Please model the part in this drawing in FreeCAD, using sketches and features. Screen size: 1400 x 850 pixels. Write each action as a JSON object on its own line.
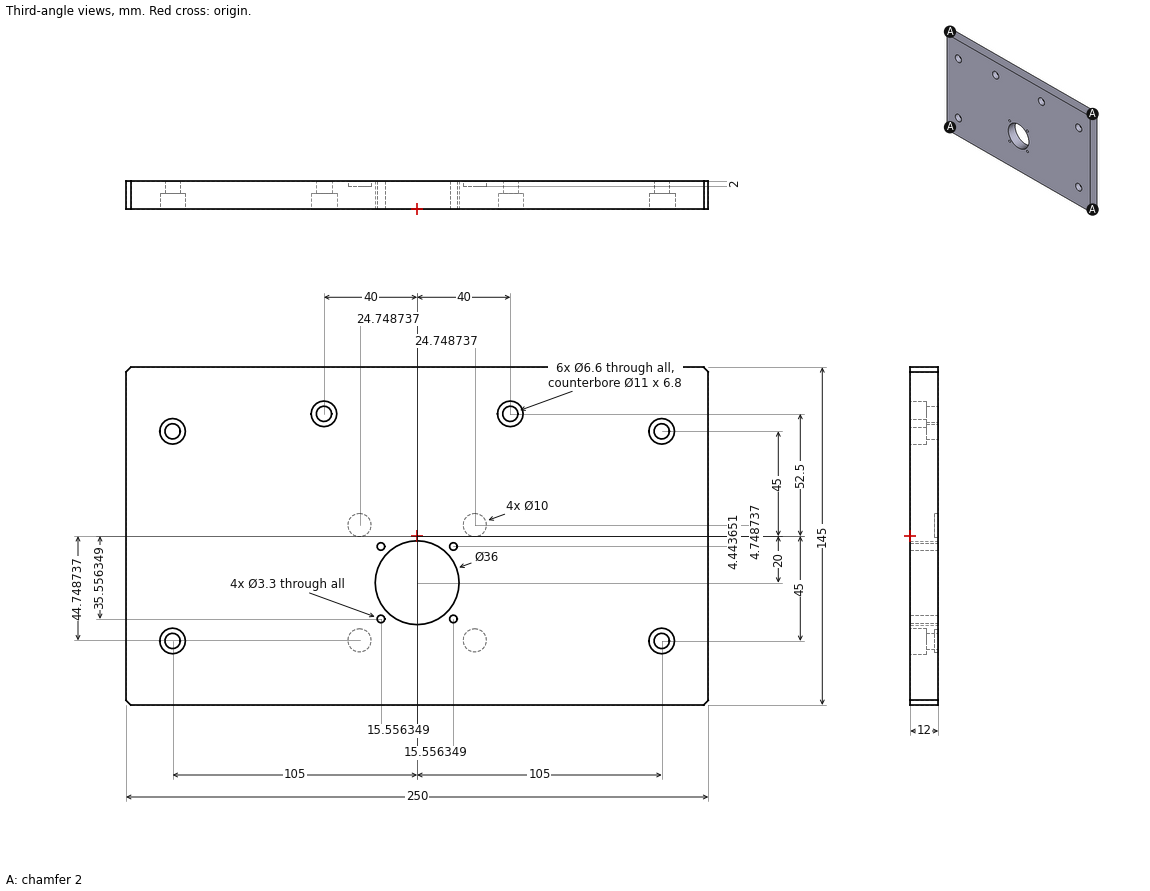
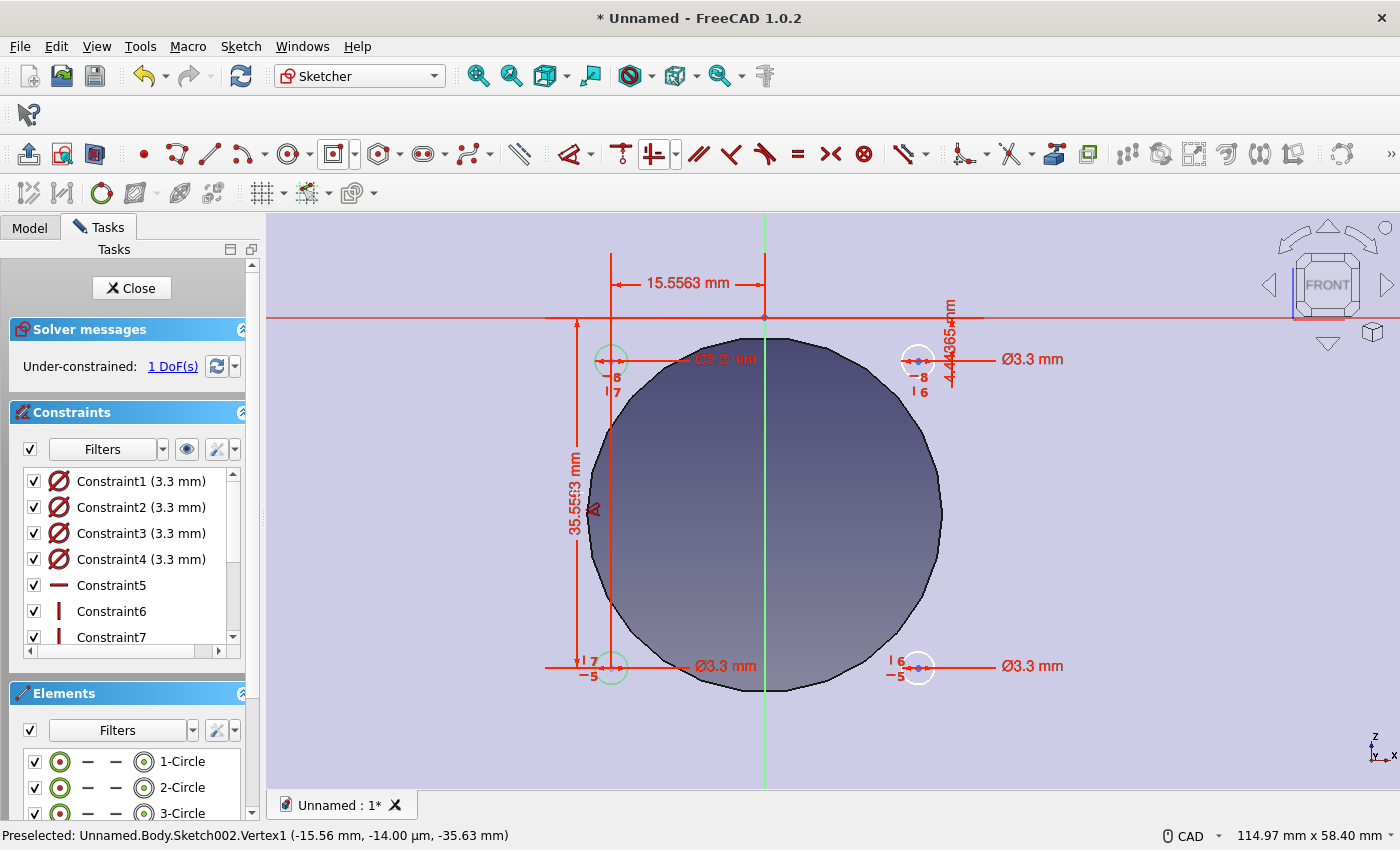
{"action": "left_click", "coordinate": [918, 668]}
{"action": "left_click", "coordinate": [841, 284]}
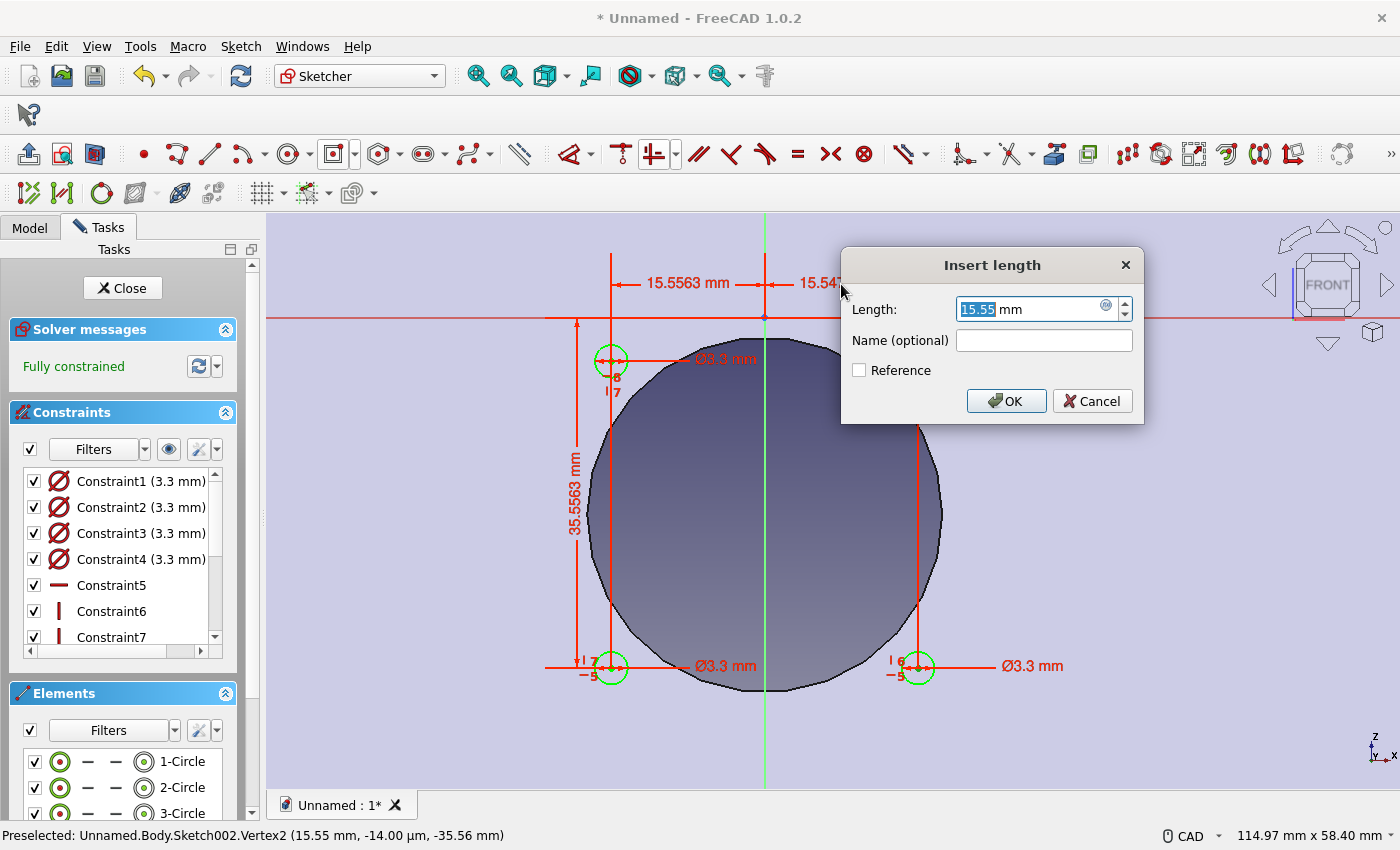
{"action": "type", "text": "15.556349"}
{"action": "key", "text": "Return"}
{"action": "key", "text": "Escape"}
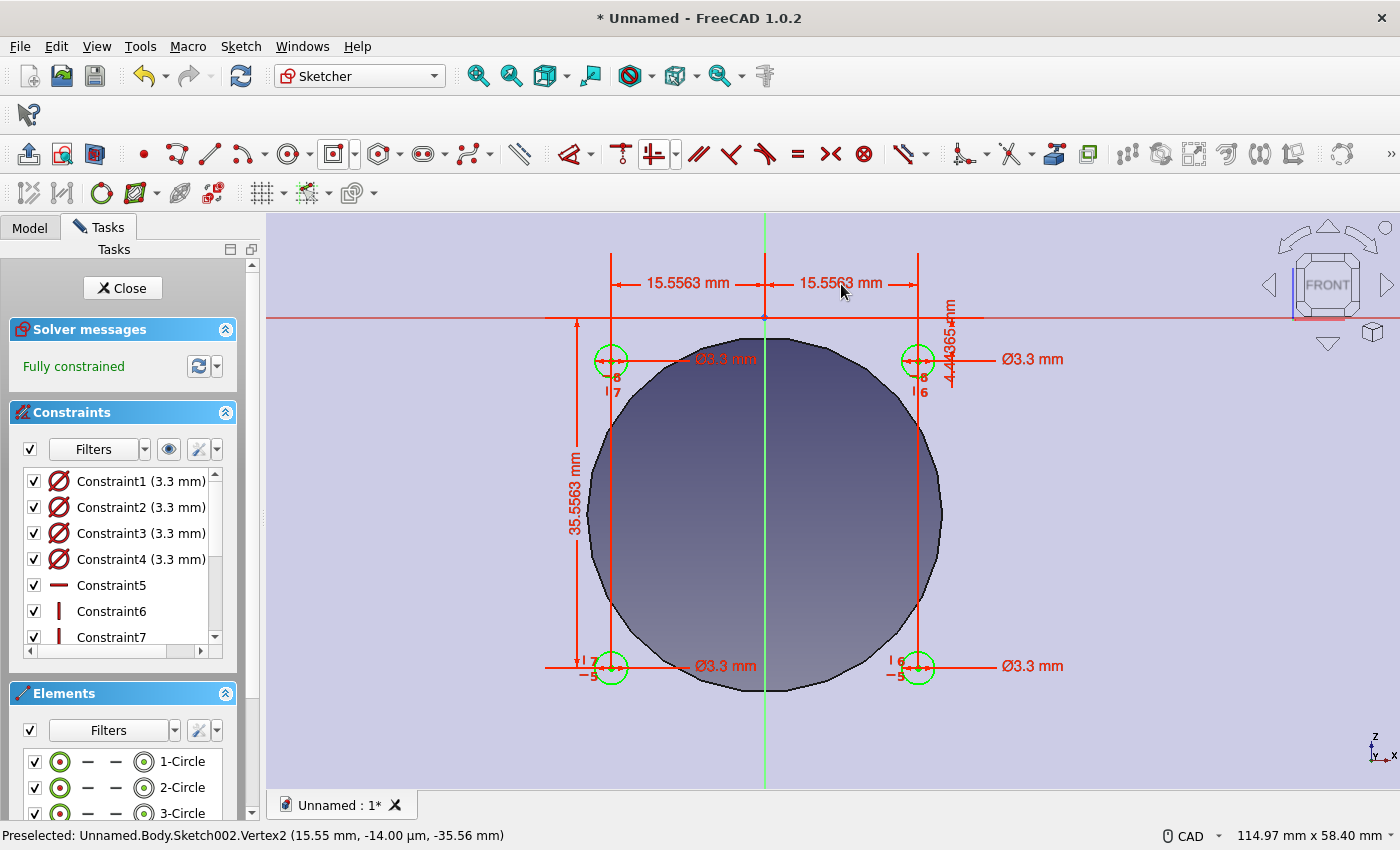
{"action": "left_click", "coordinate": [123, 288]}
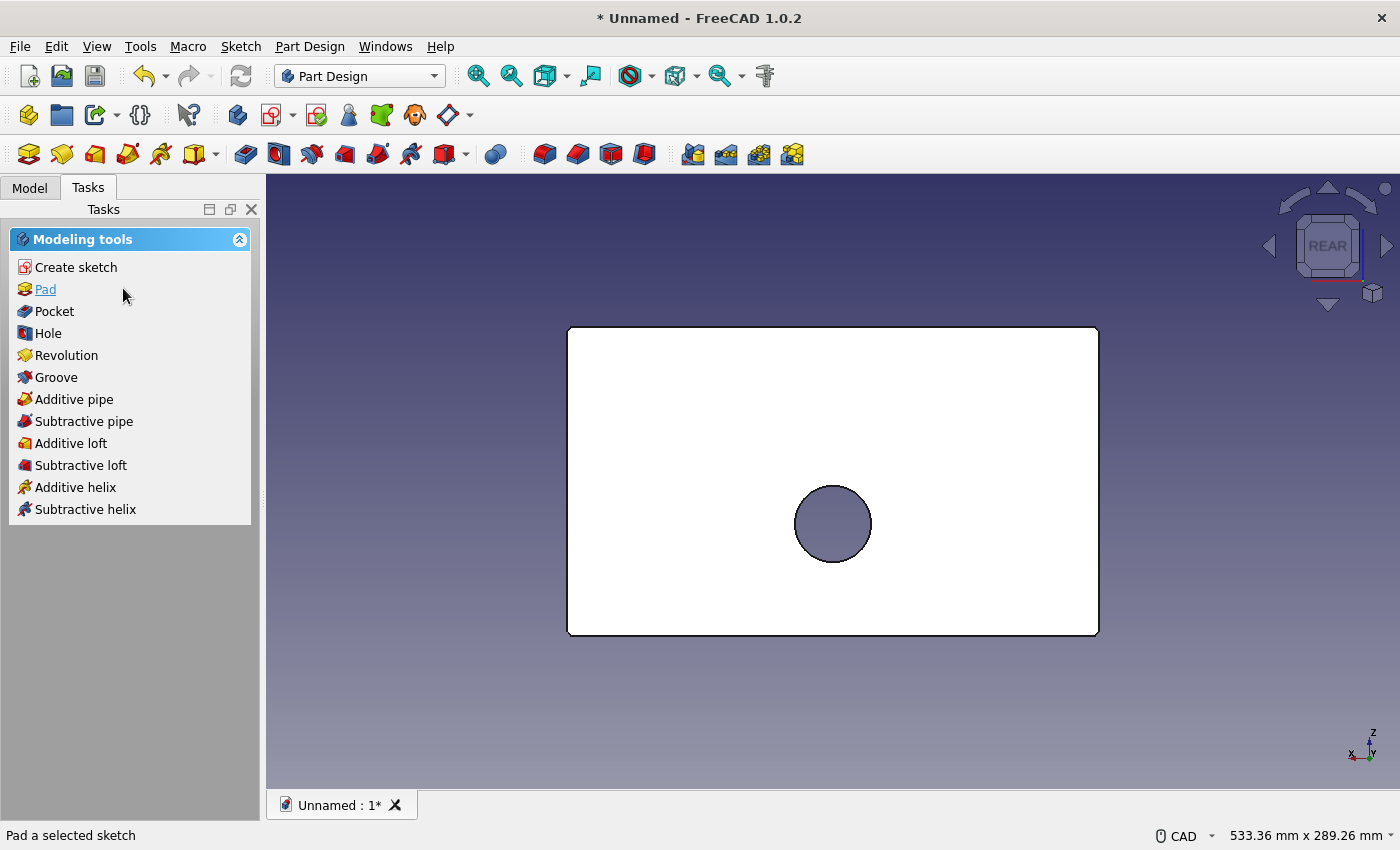
{"action": "left_click", "coordinate": [279, 154]}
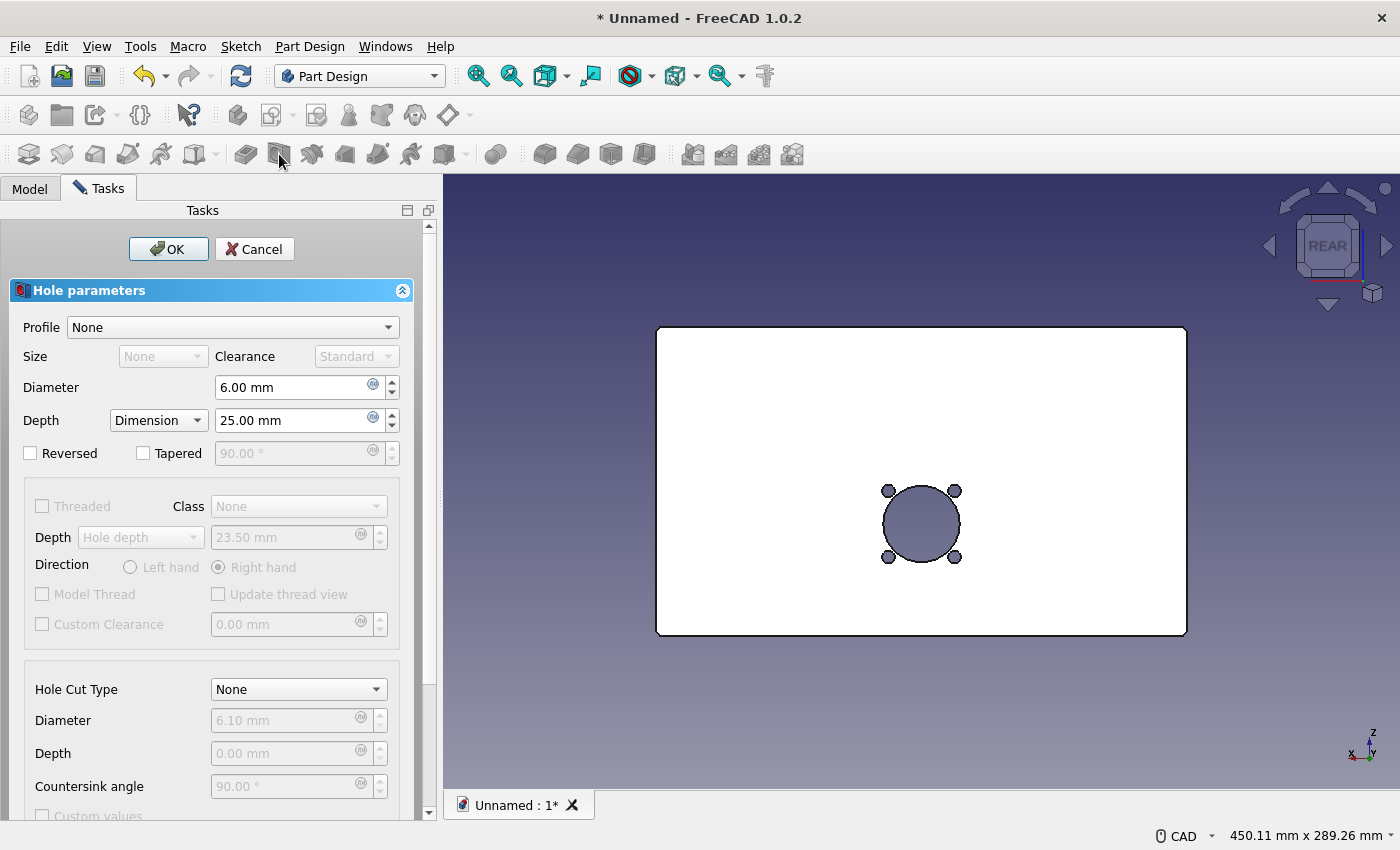
{"action": "triple_click", "coordinate": [300, 388]}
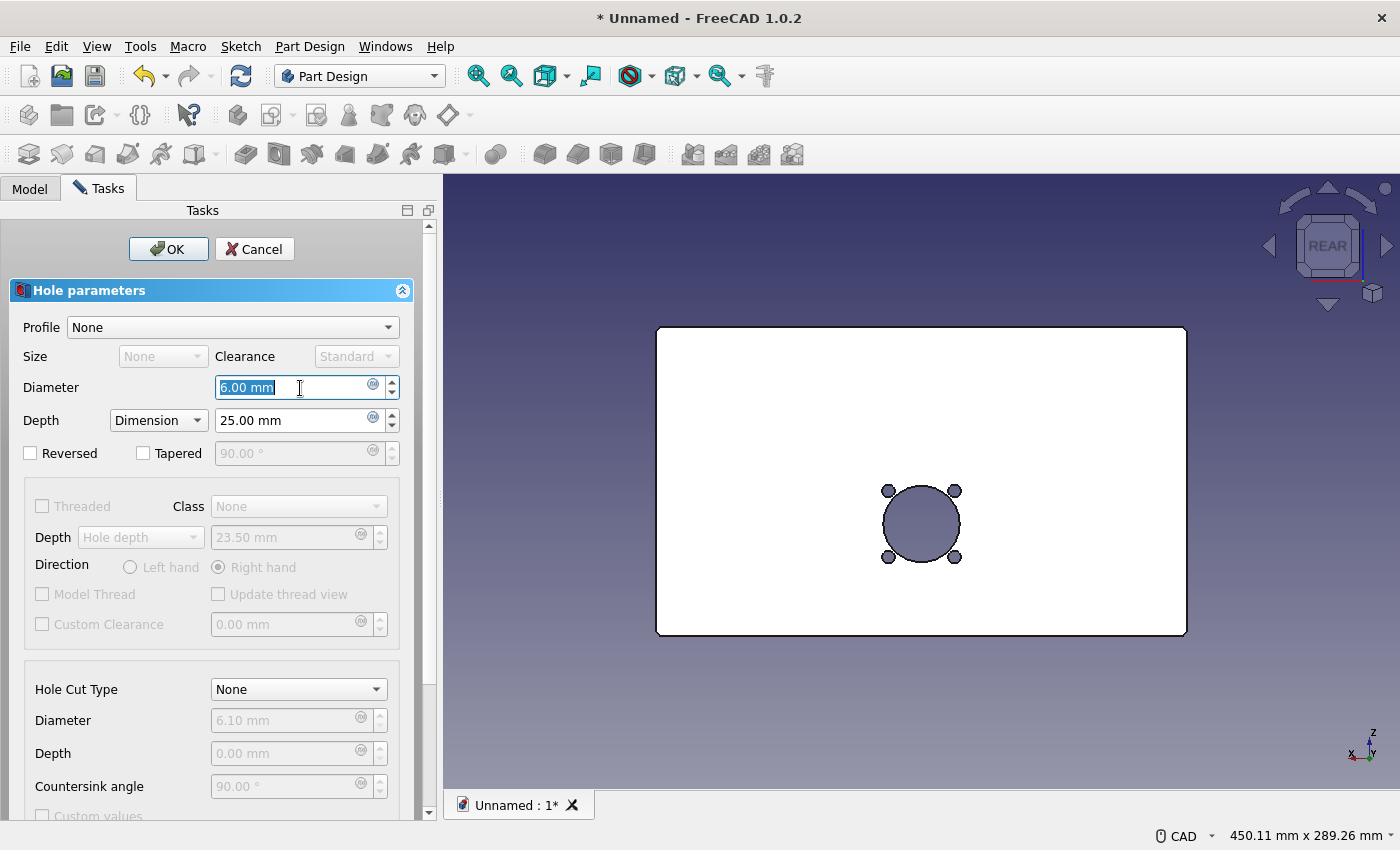
{"action": "type", "text": "3.3"}
{"action": "key", "text": "Tab"}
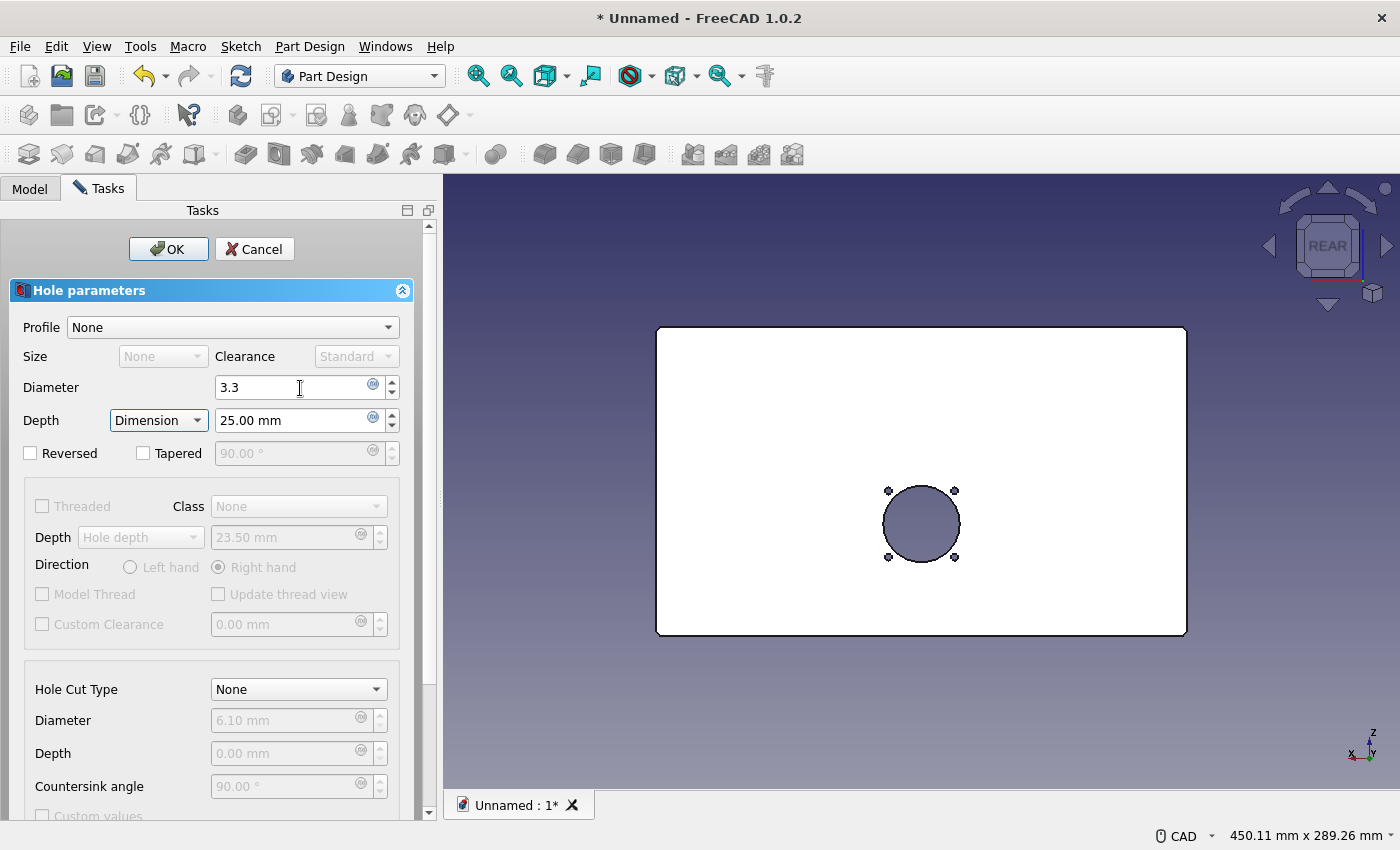
{"action": "left_click", "coordinate": [160, 420]}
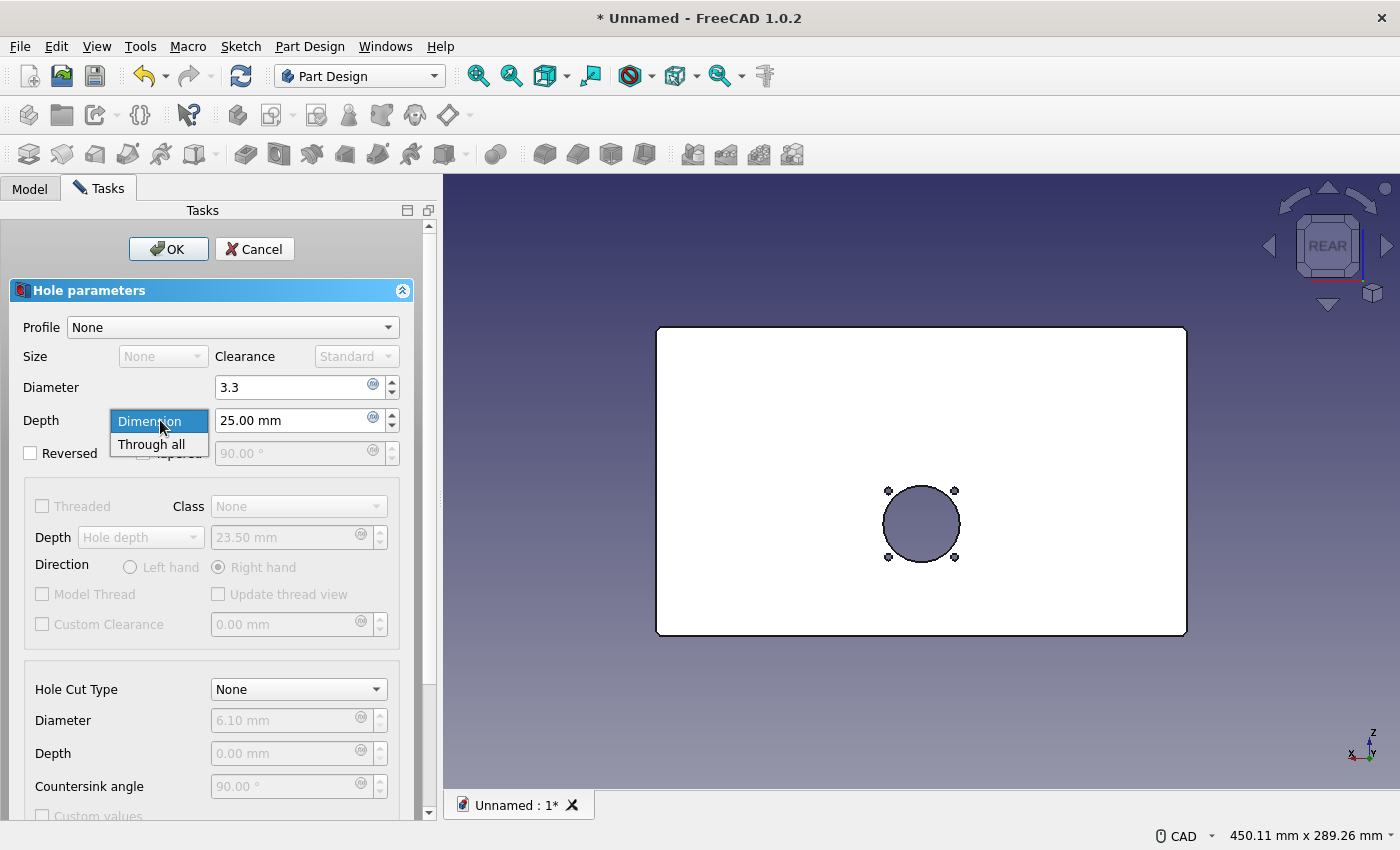
{"action": "left_click", "coordinate": [158, 444]}